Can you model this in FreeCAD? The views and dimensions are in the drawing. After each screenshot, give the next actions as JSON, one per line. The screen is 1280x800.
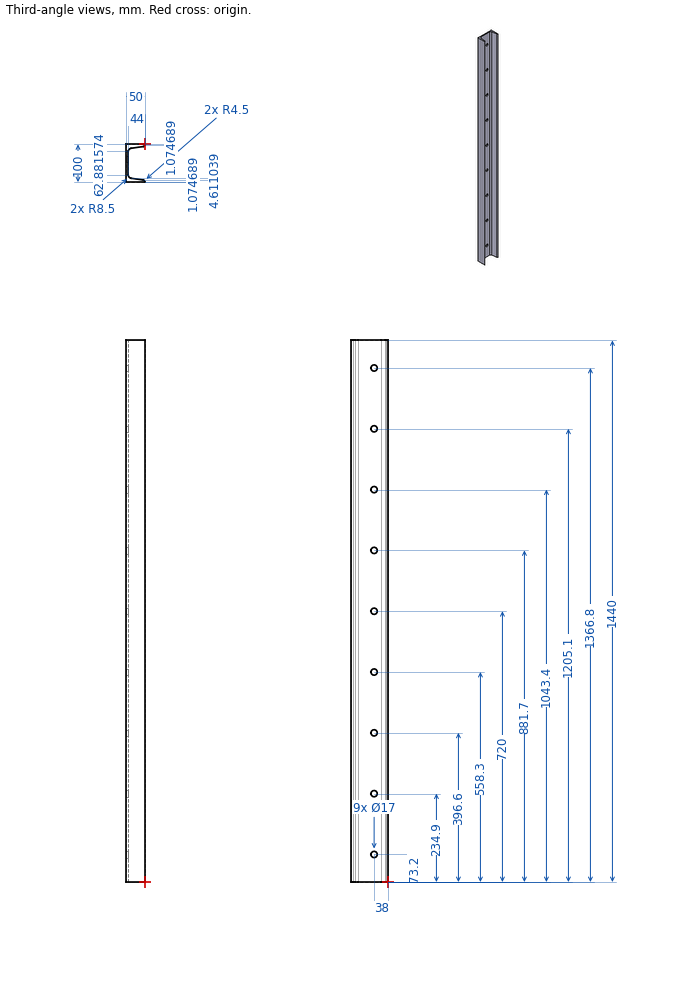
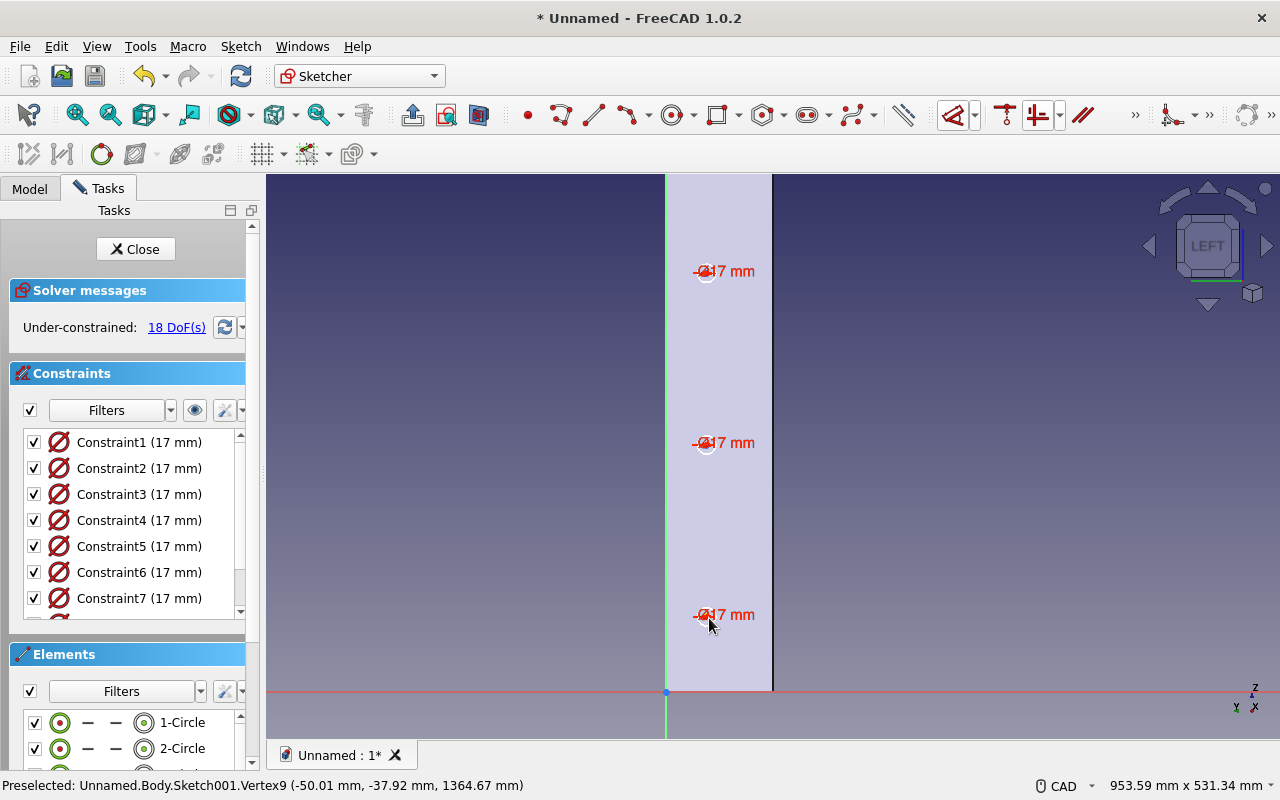
{"action": "left_click", "coordinate": [707, 617]}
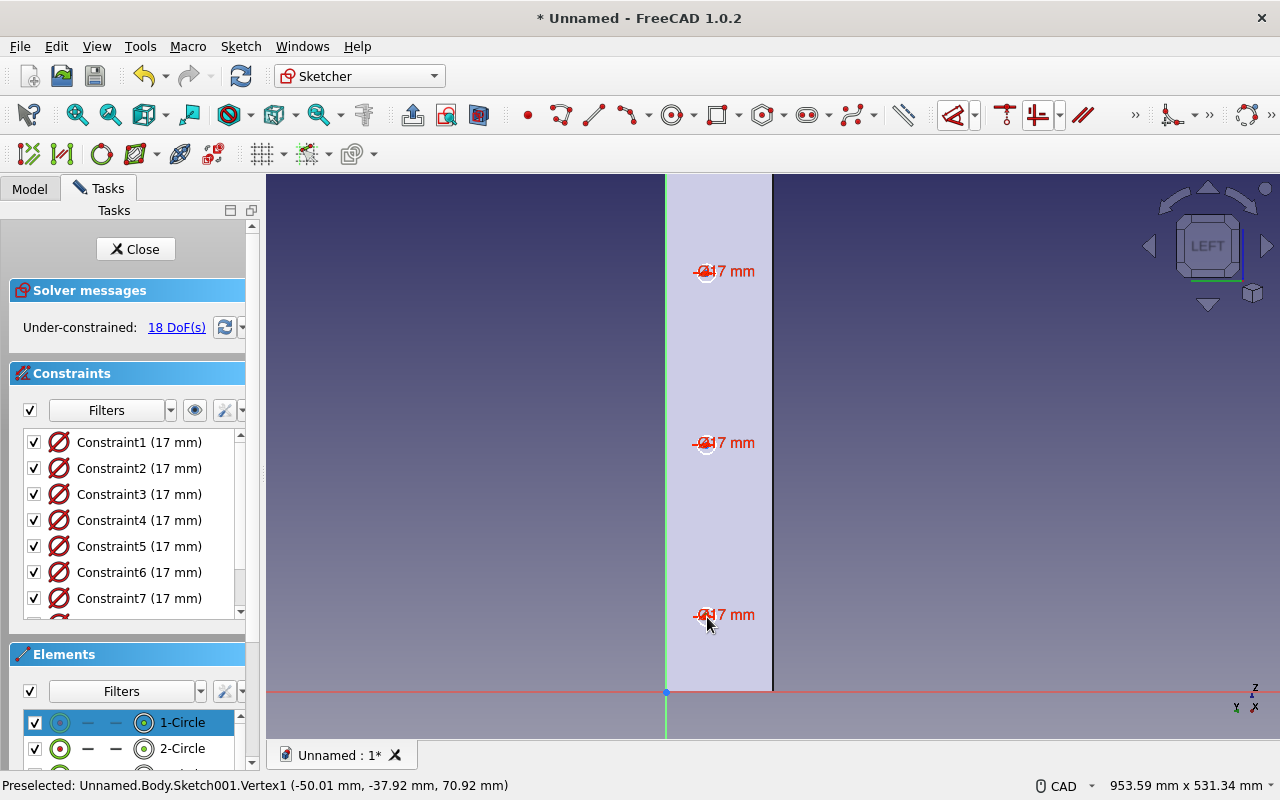
{"action": "left_click", "coordinate": [974, 116]}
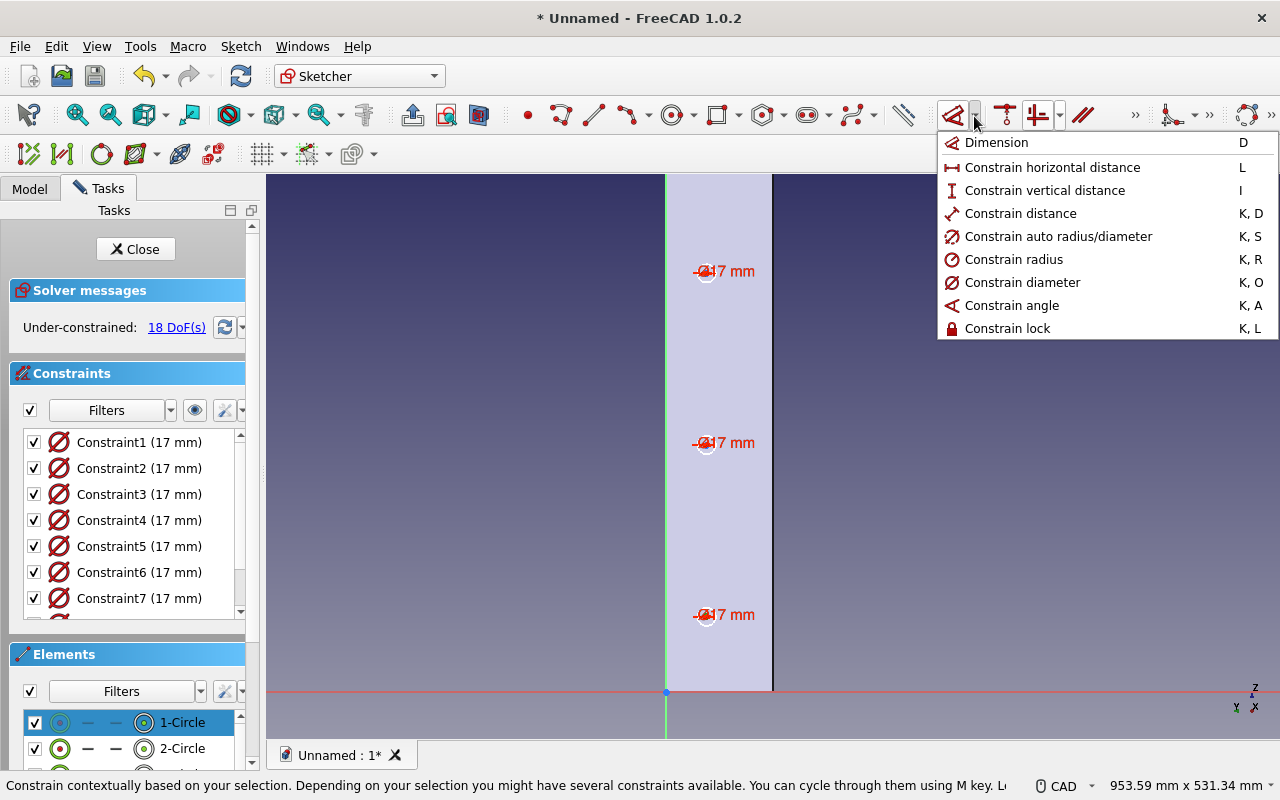
{"action": "left_click", "coordinate": [1108, 168]}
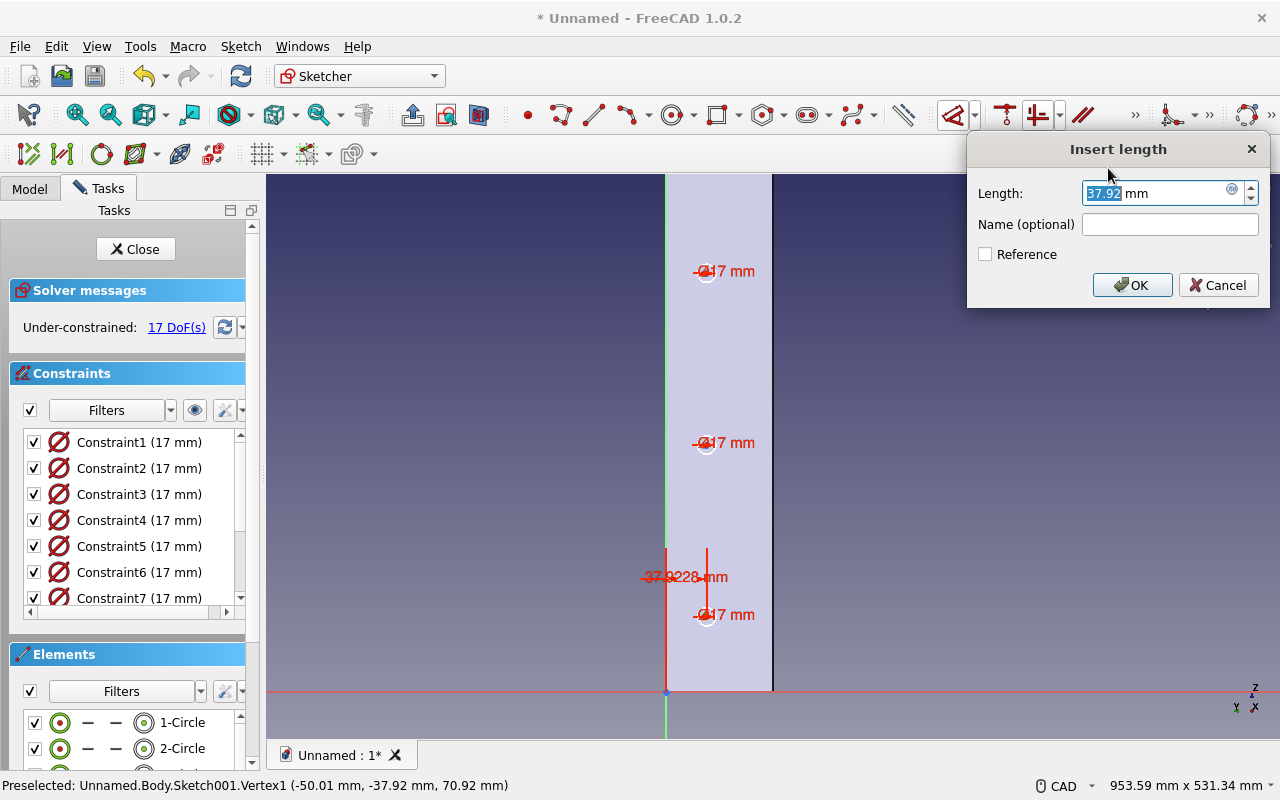
{"action": "type", "text": "38"}
{"action": "key", "text": "Return"}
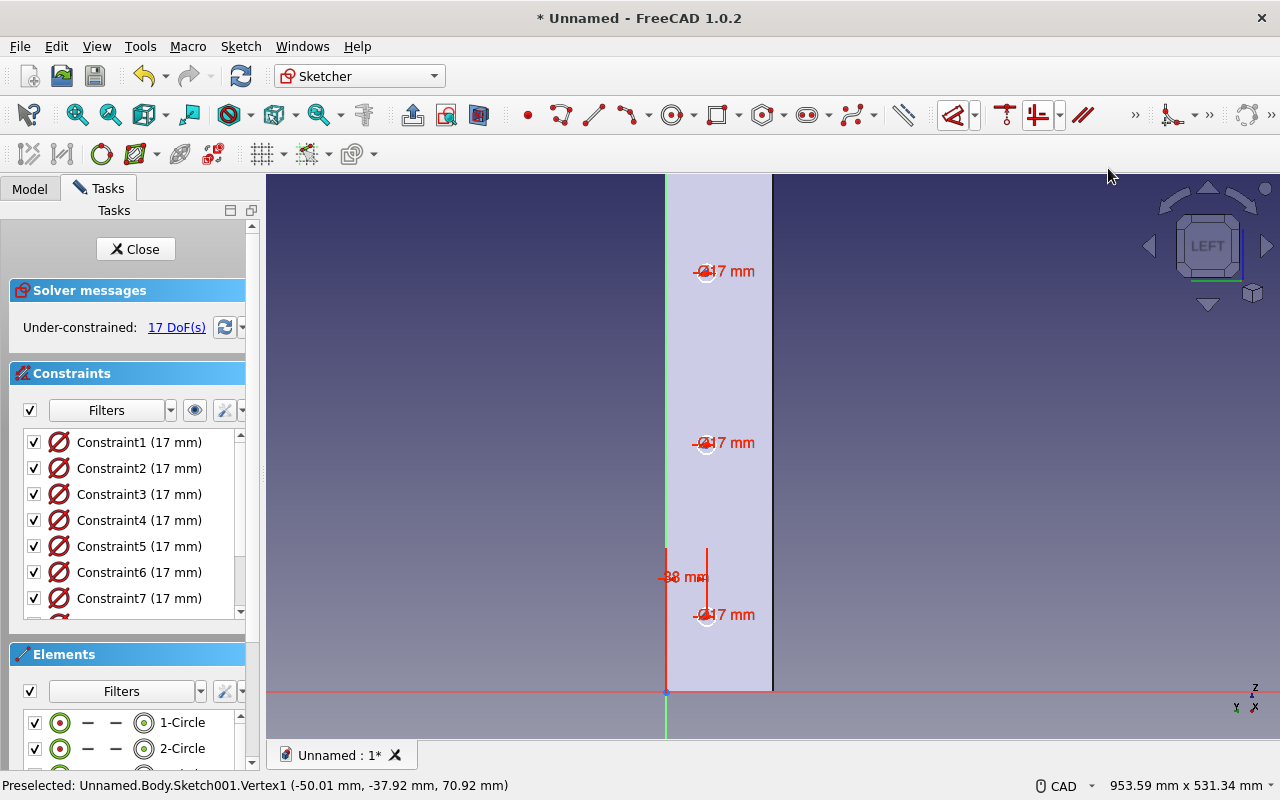
{"action": "left_click", "coordinate": [707, 445]}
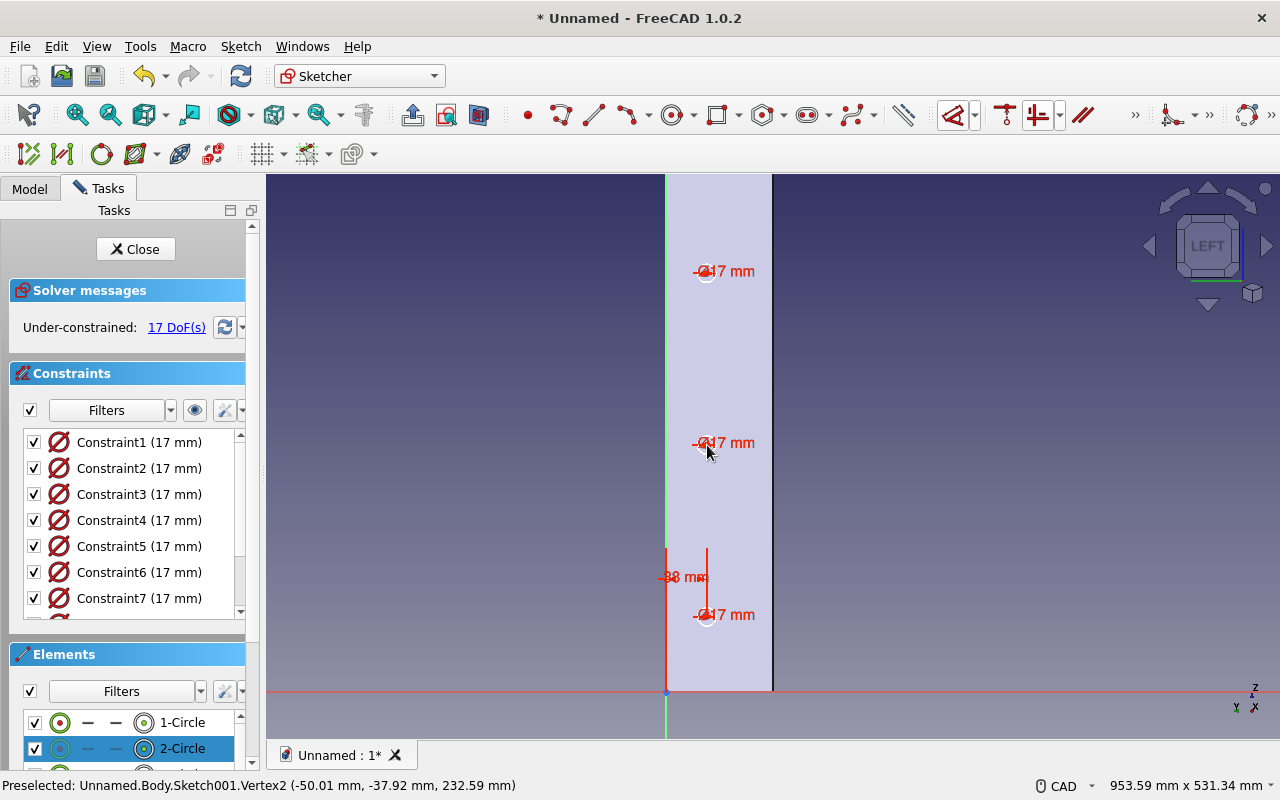
{"action": "left_click", "coordinate": [974, 116]}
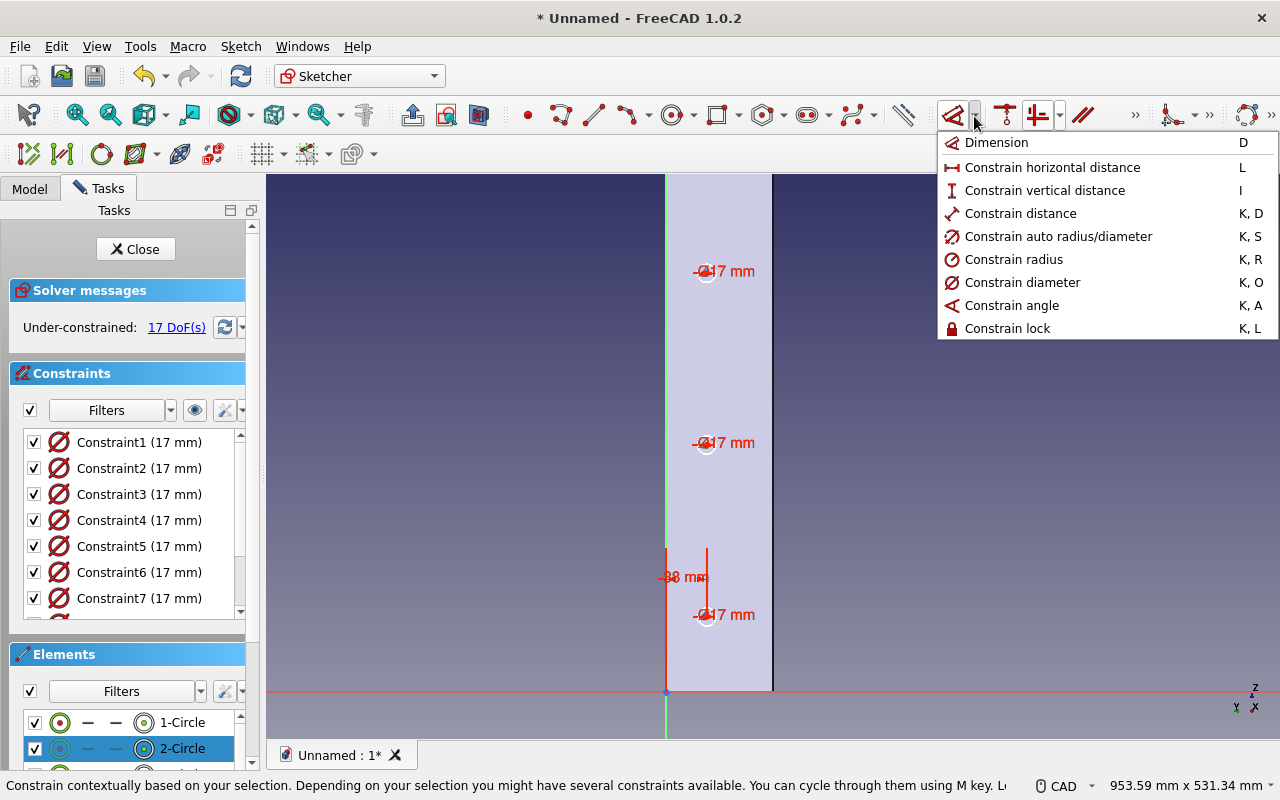
{"action": "left_click", "coordinate": [1108, 168]}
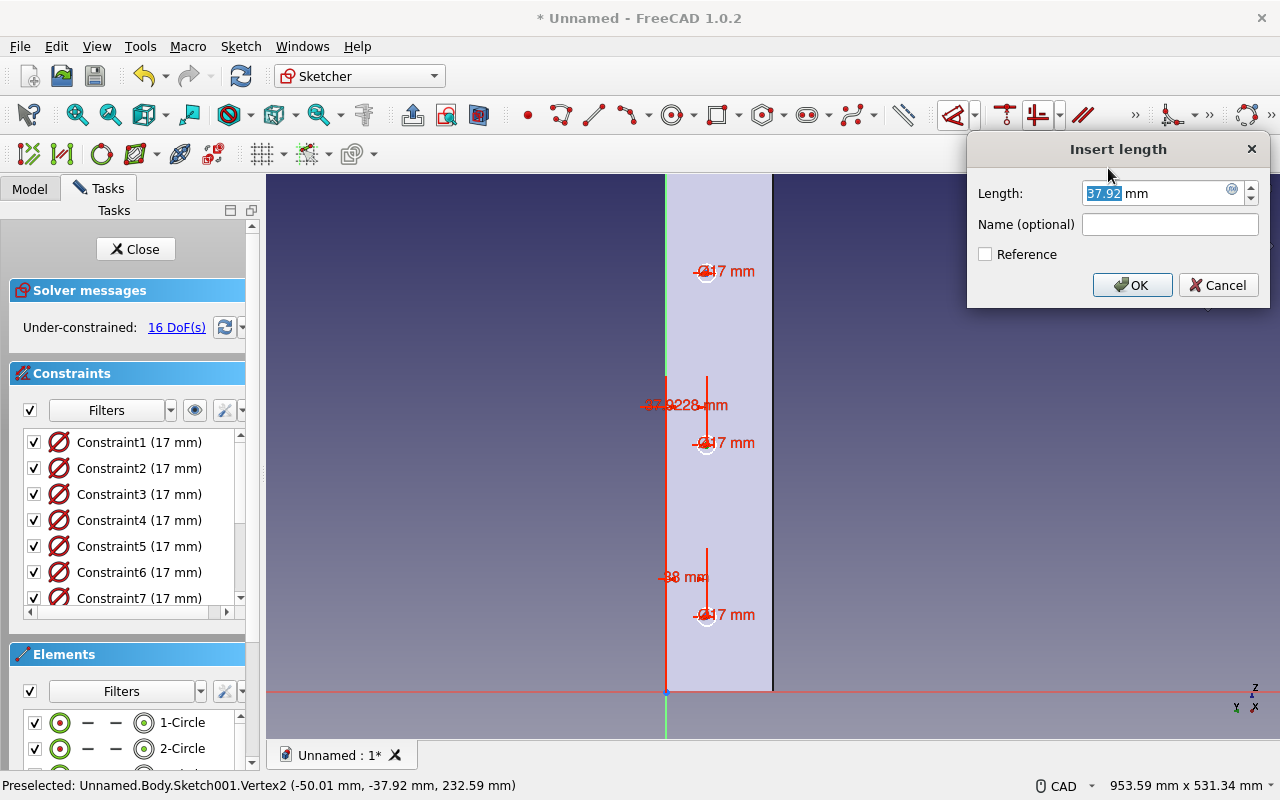
{"action": "type", "text": "38"}
{"action": "key", "text": "Return"}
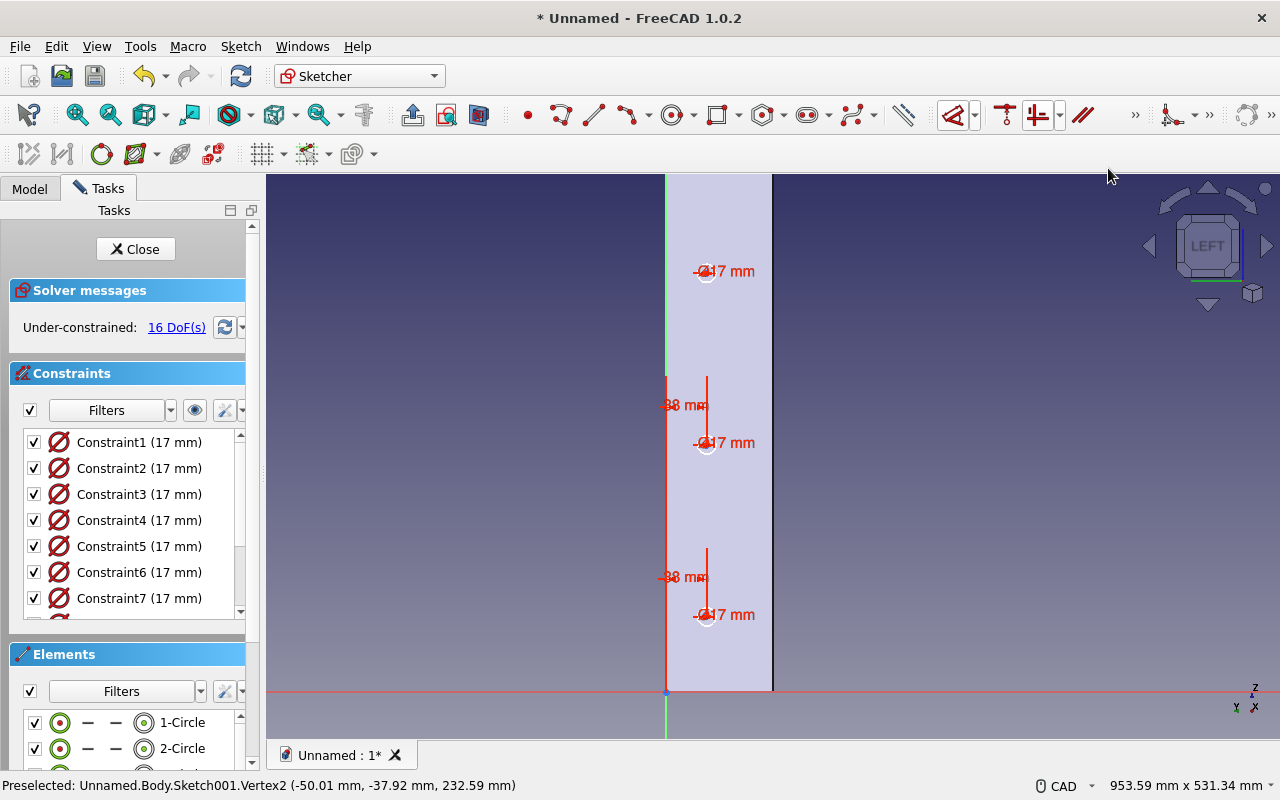
{"action": "left_click", "coordinate": [707, 273]}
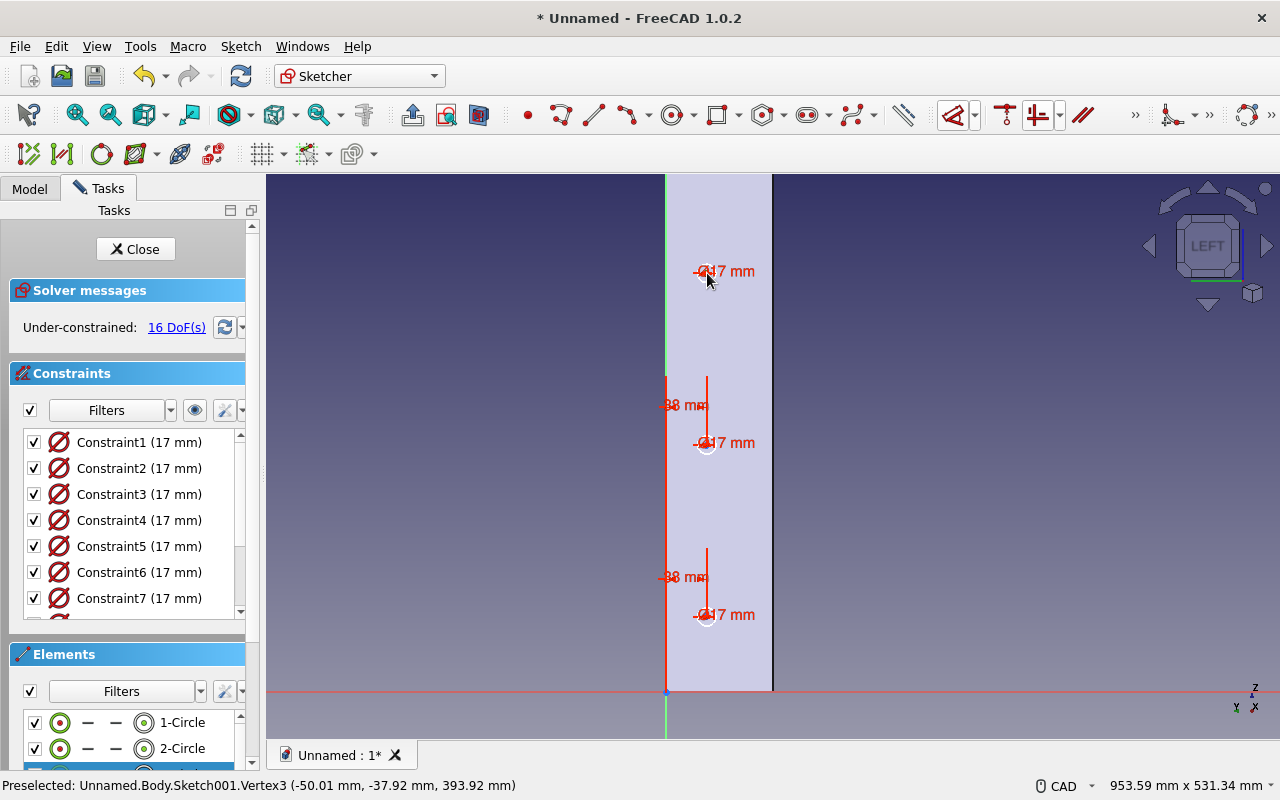
{"action": "left_click", "coordinate": [974, 116]}